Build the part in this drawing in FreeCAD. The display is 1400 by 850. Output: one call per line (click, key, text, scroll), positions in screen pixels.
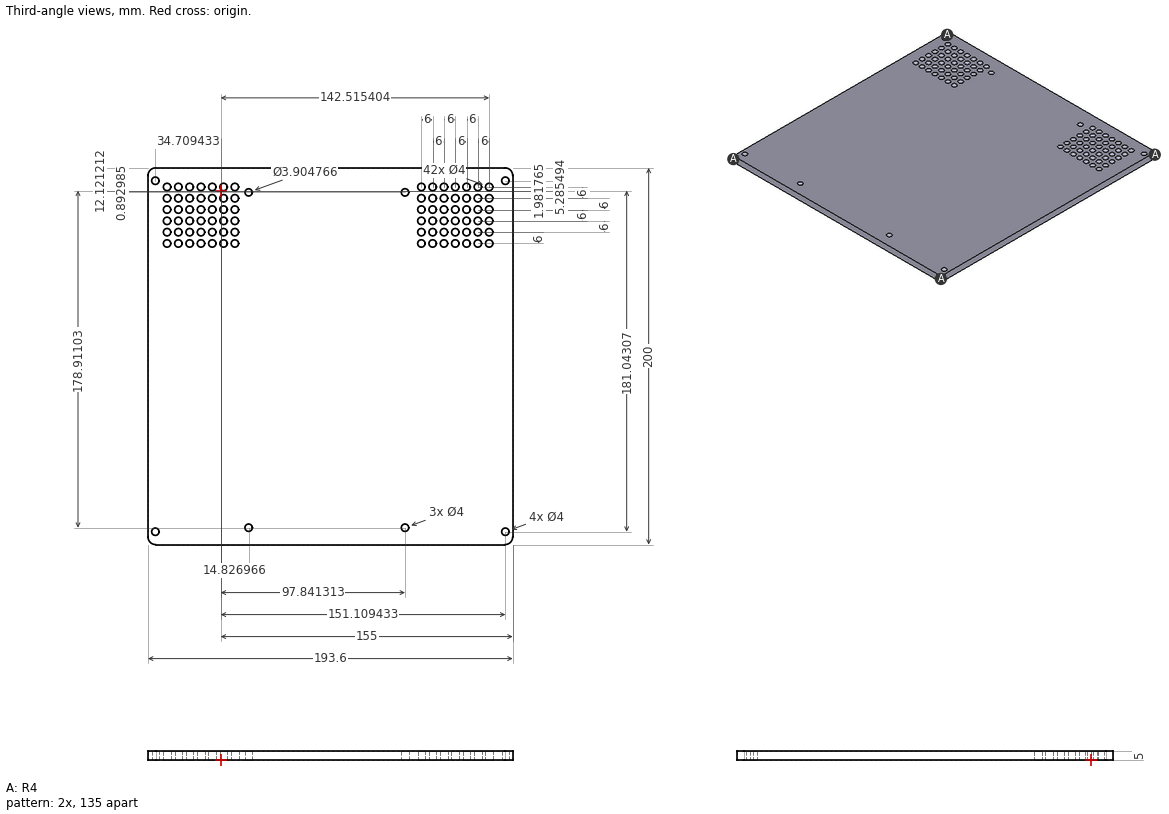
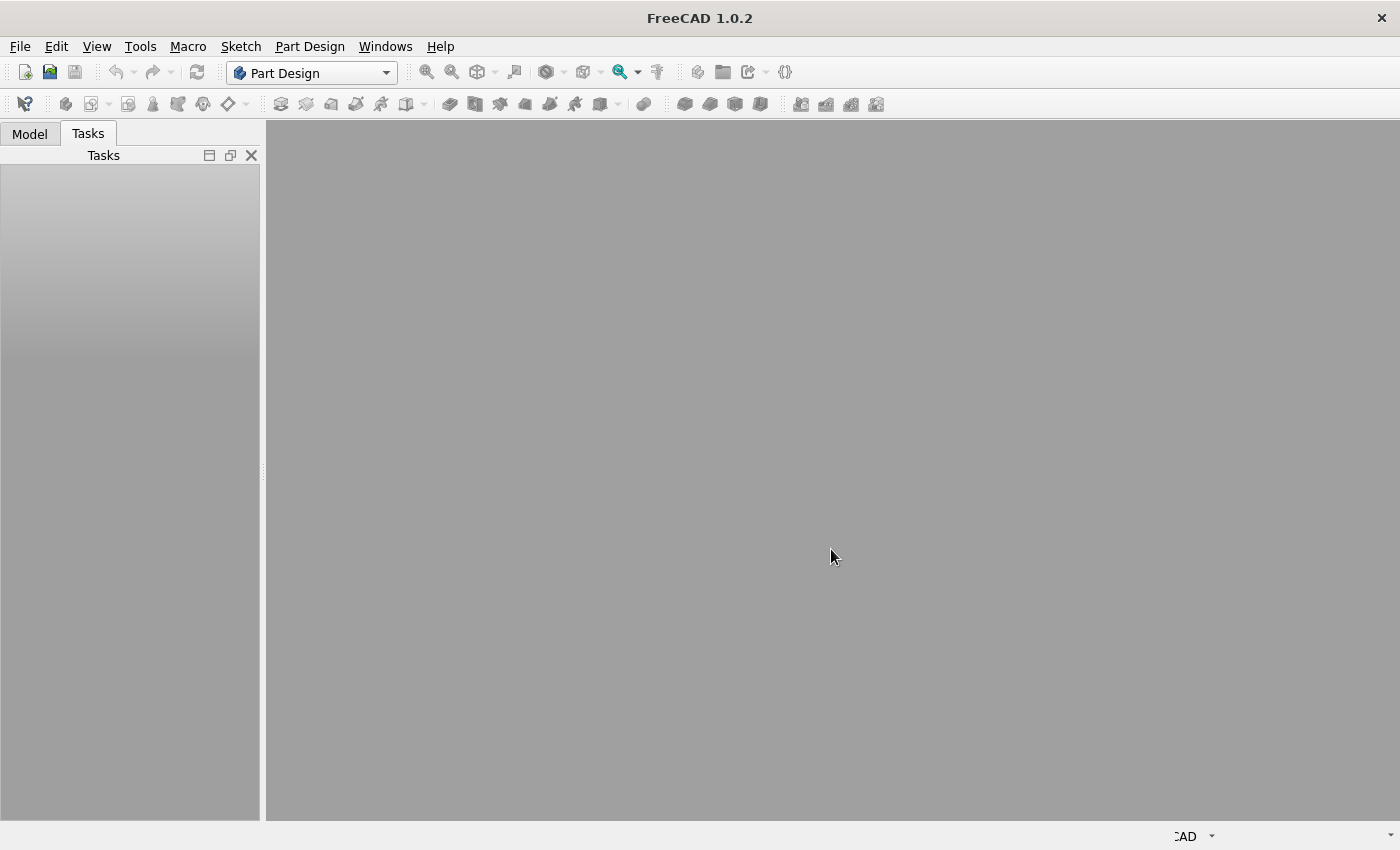
click(25, 72)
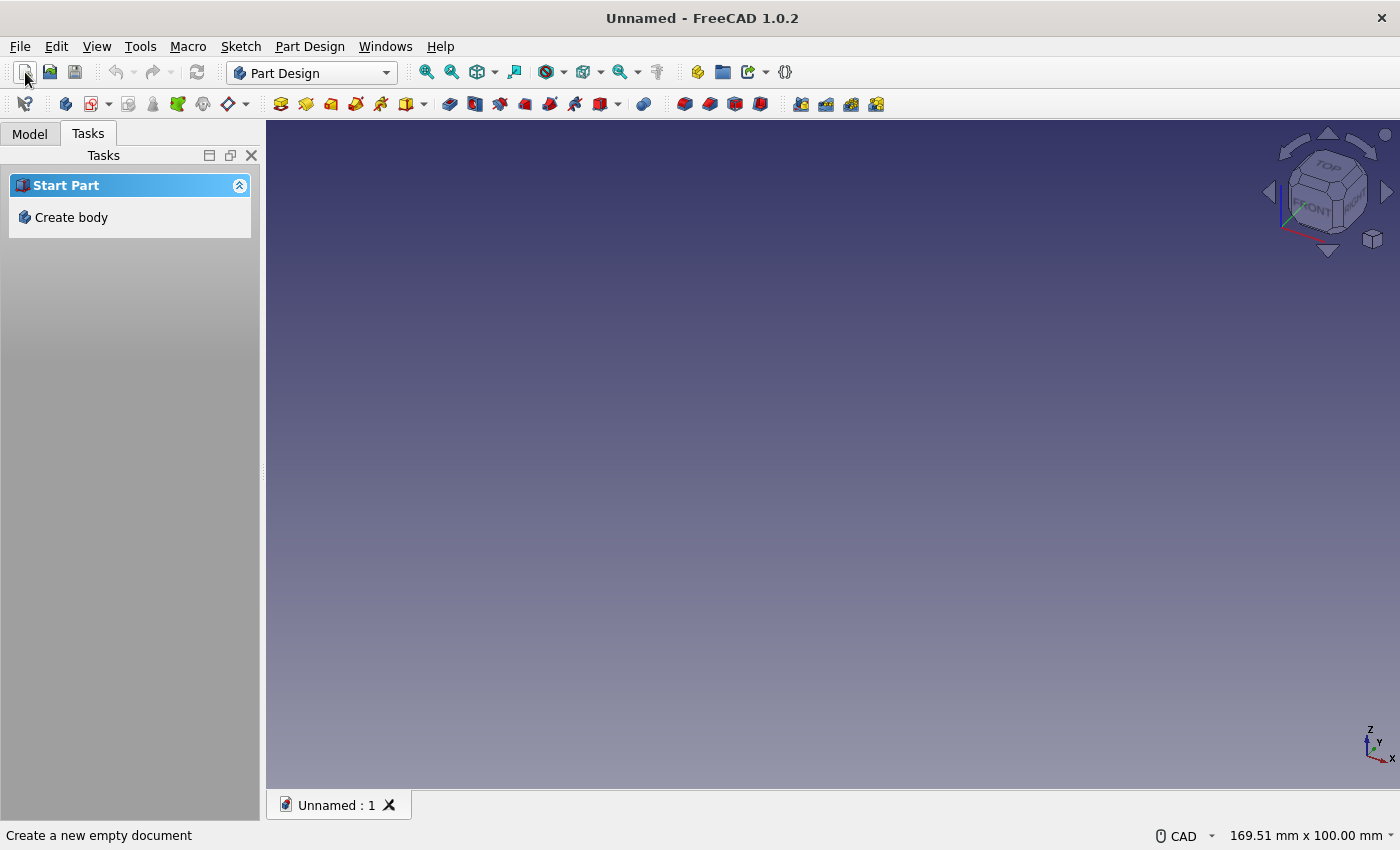
click(90, 104)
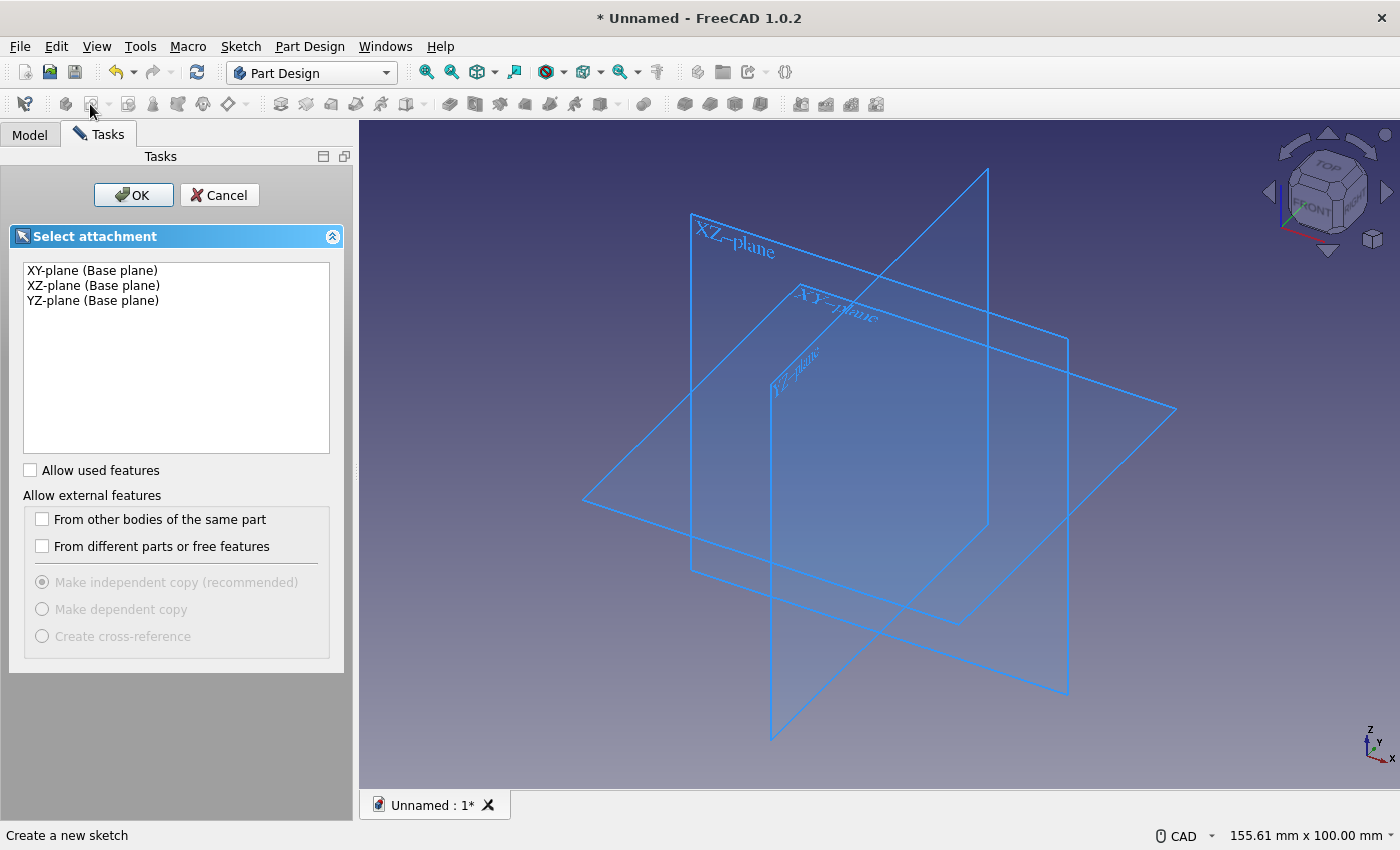
click(84, 270)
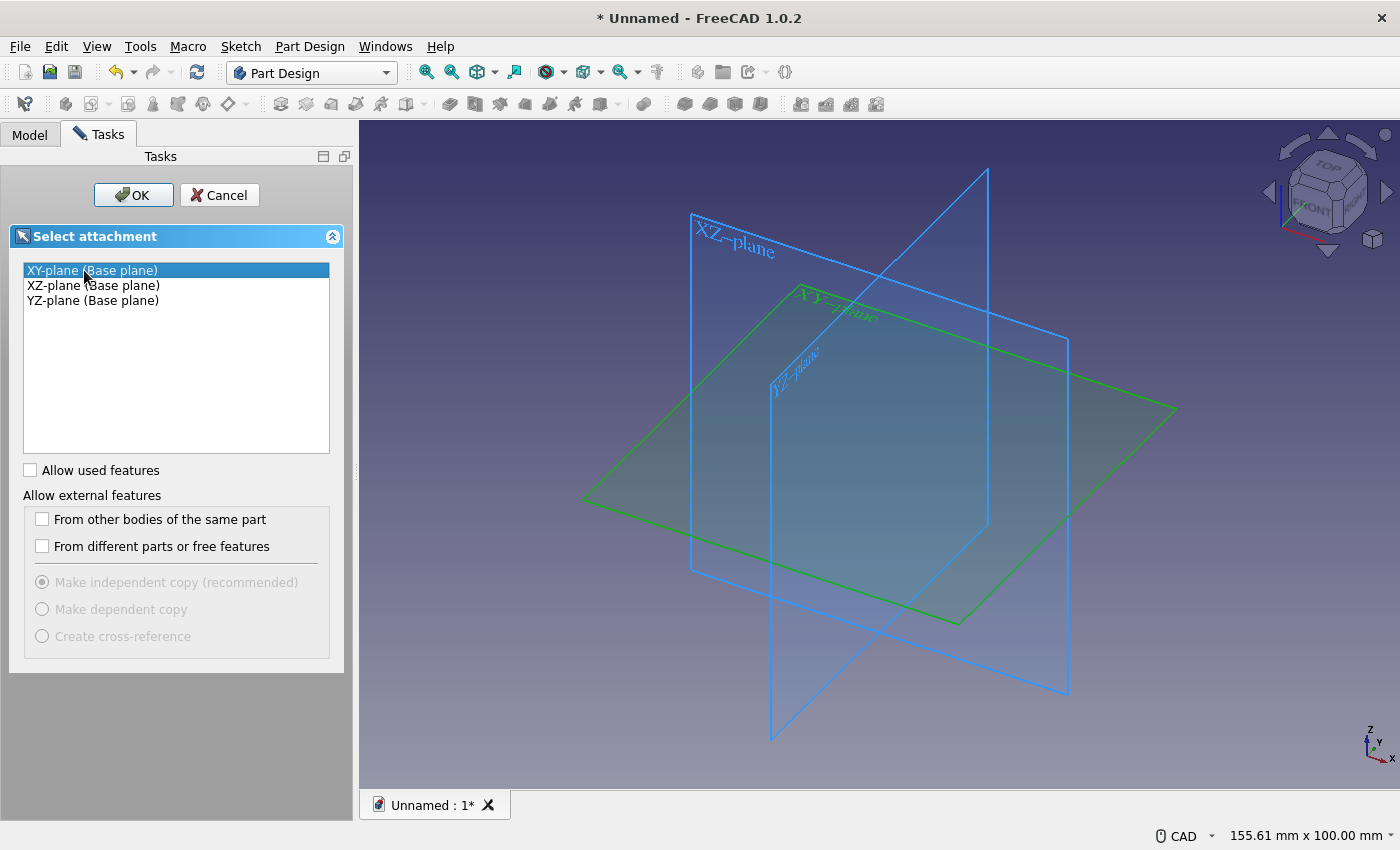
click(134, 195)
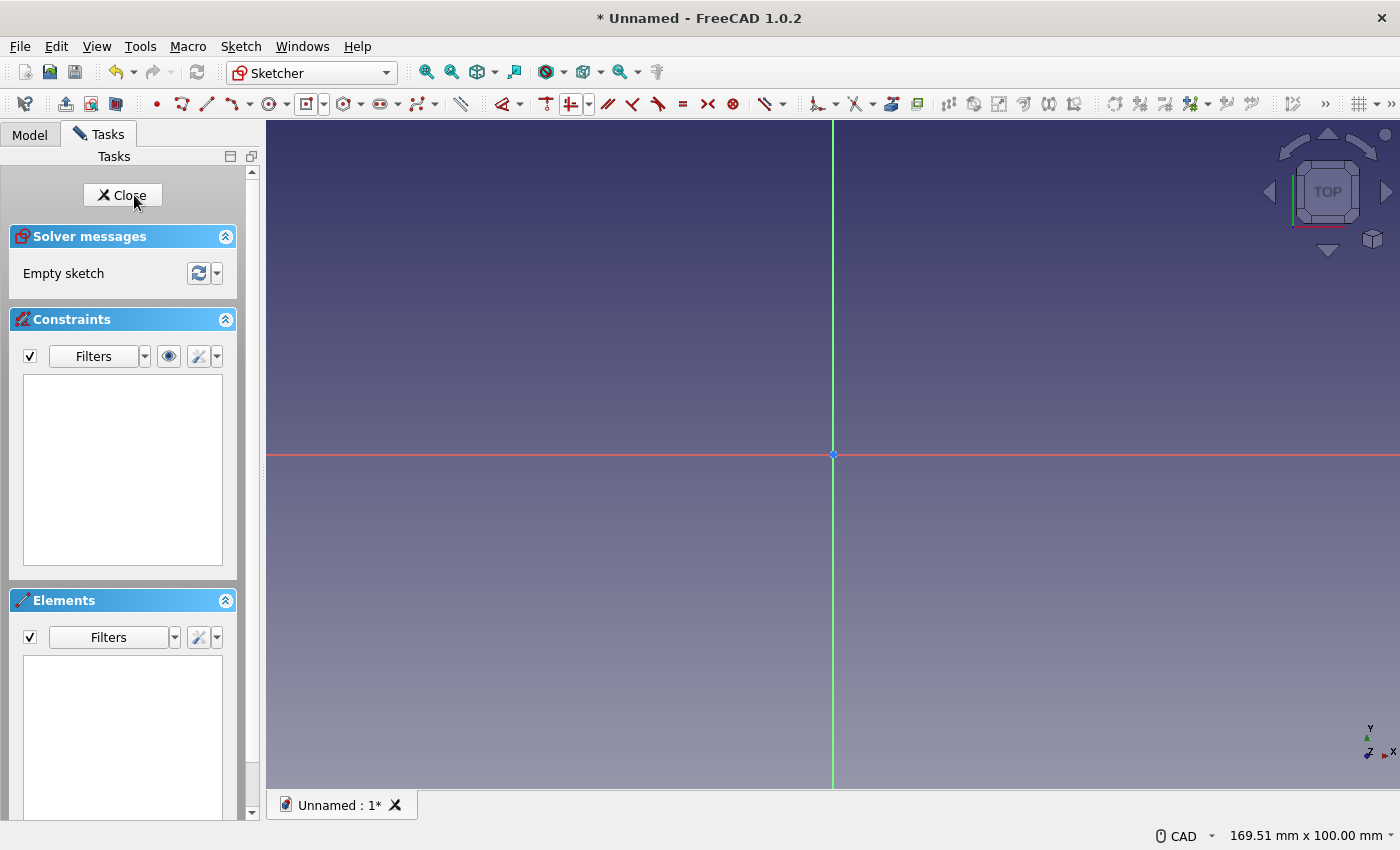
scroll(567, 201, down, 6)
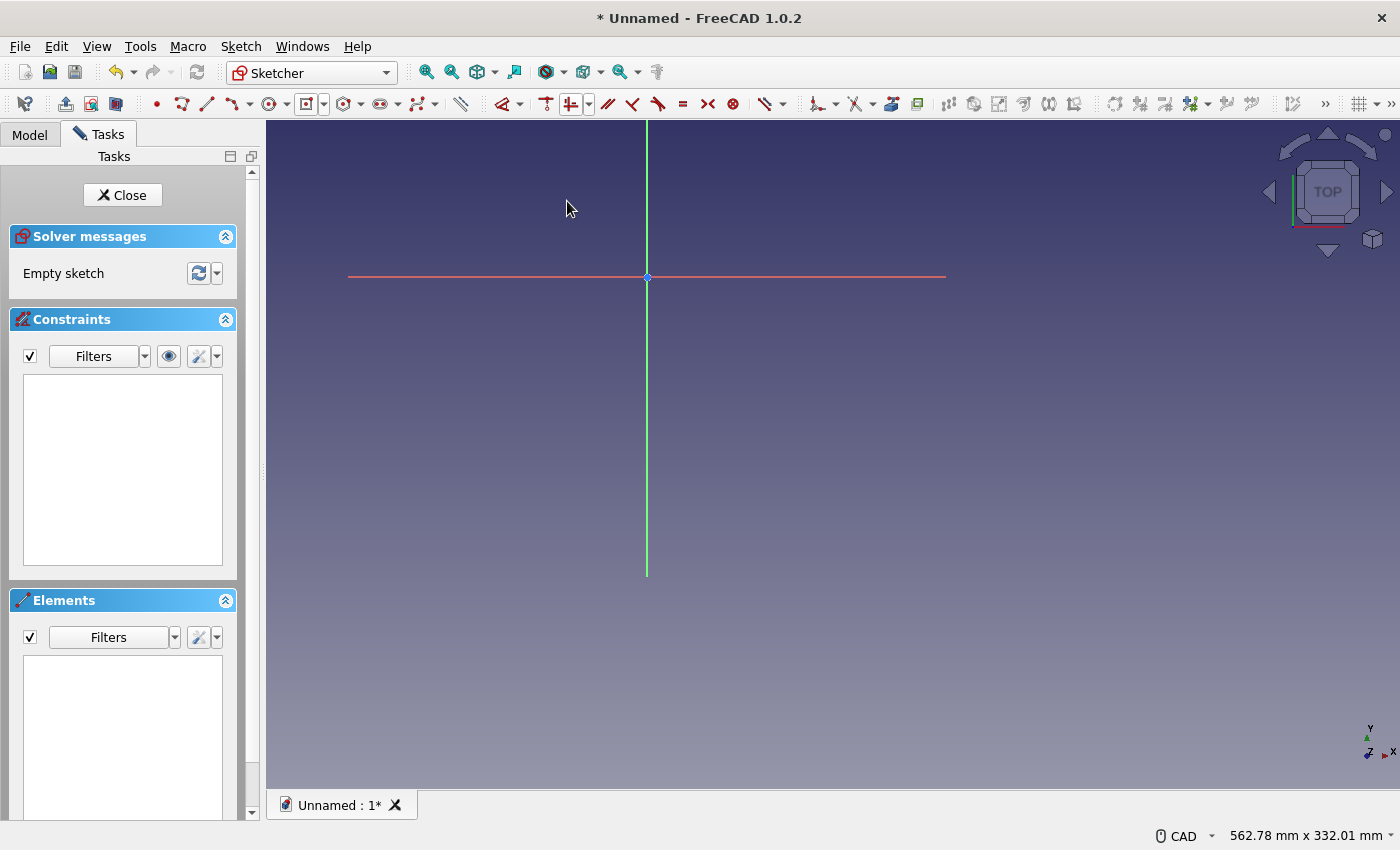
key(g)
key(r)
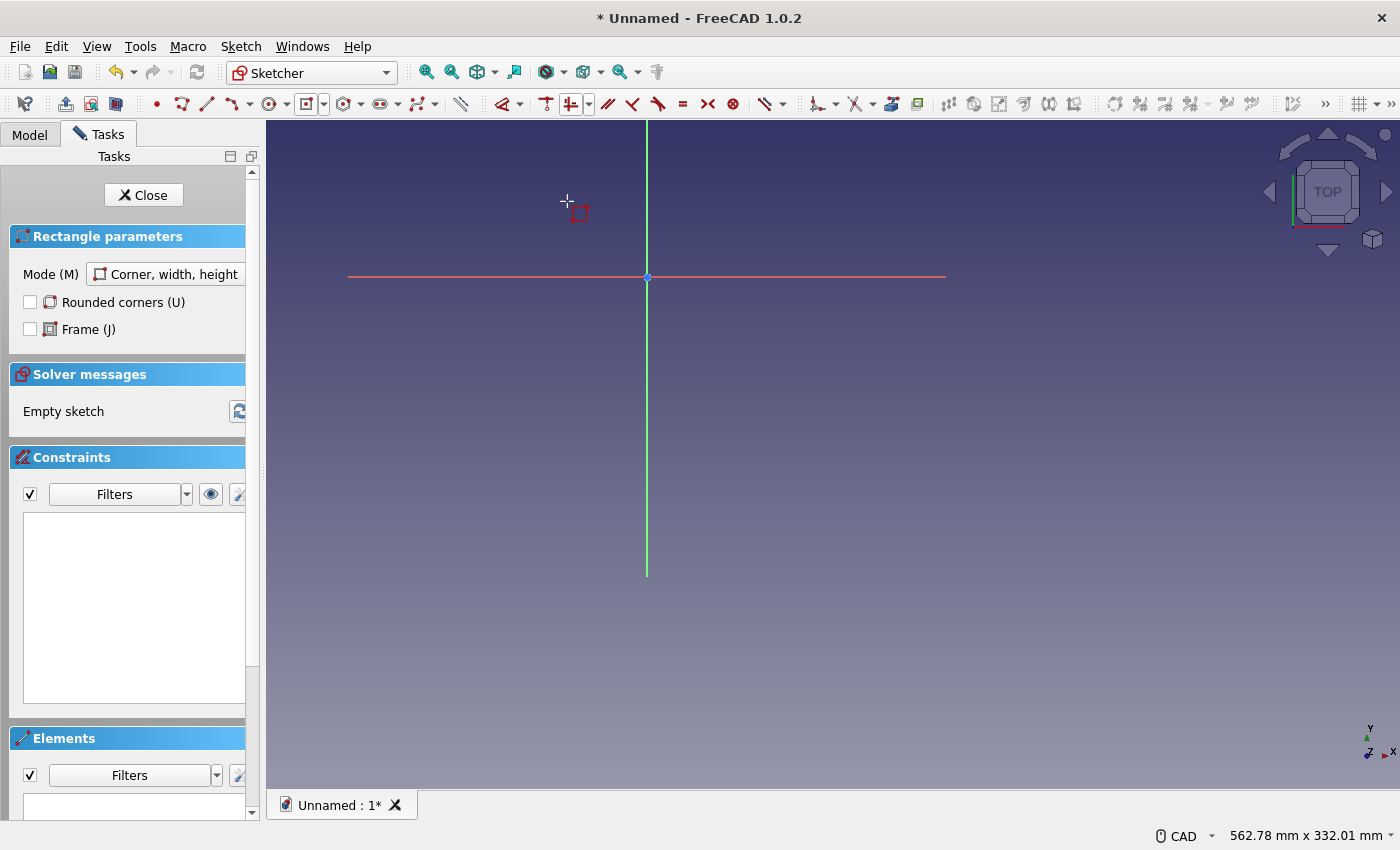
click(570, 253)
move(960, 656)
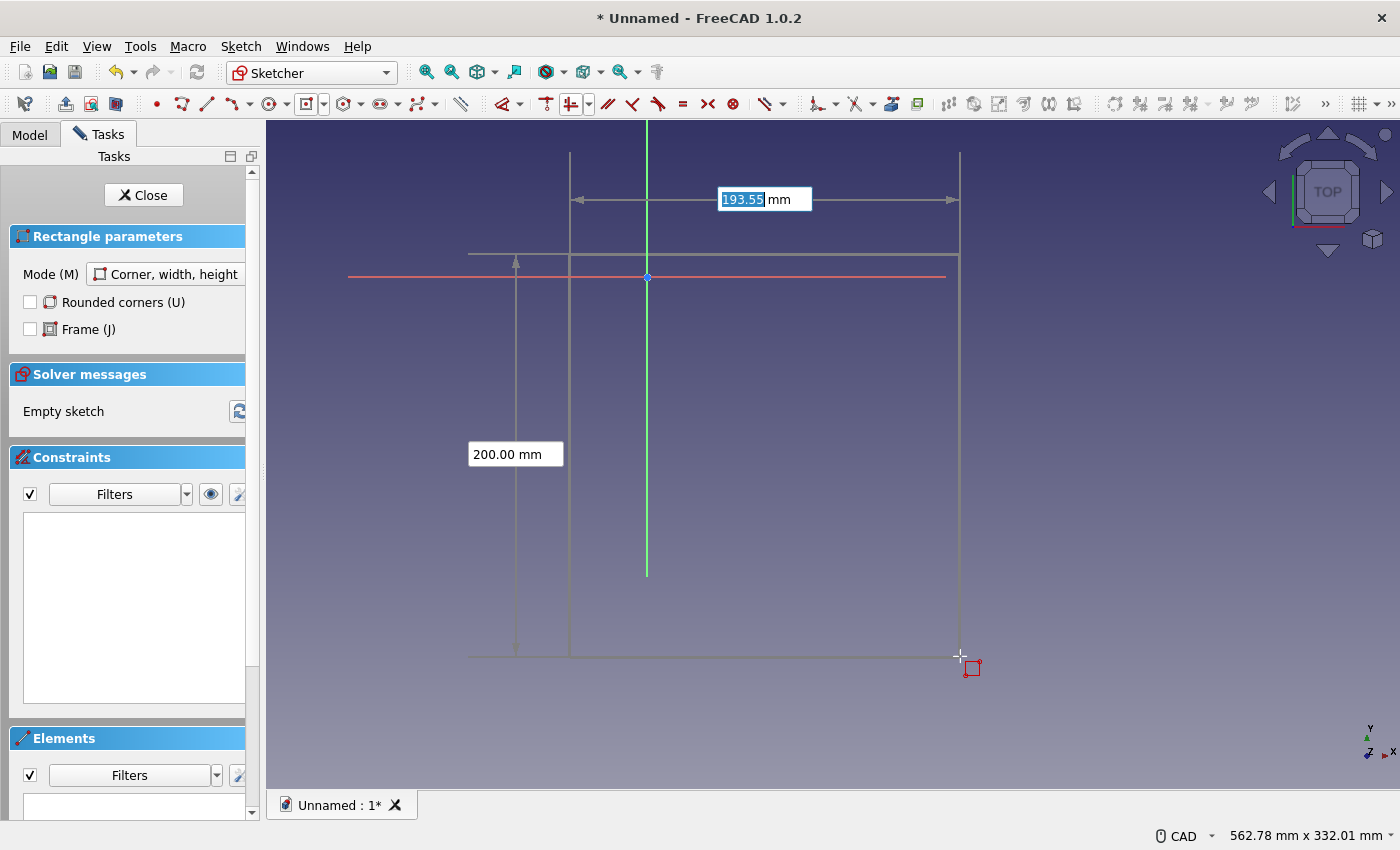
text(193.6)
key(Tab)
text(200)
key(Return)
key(Escape)